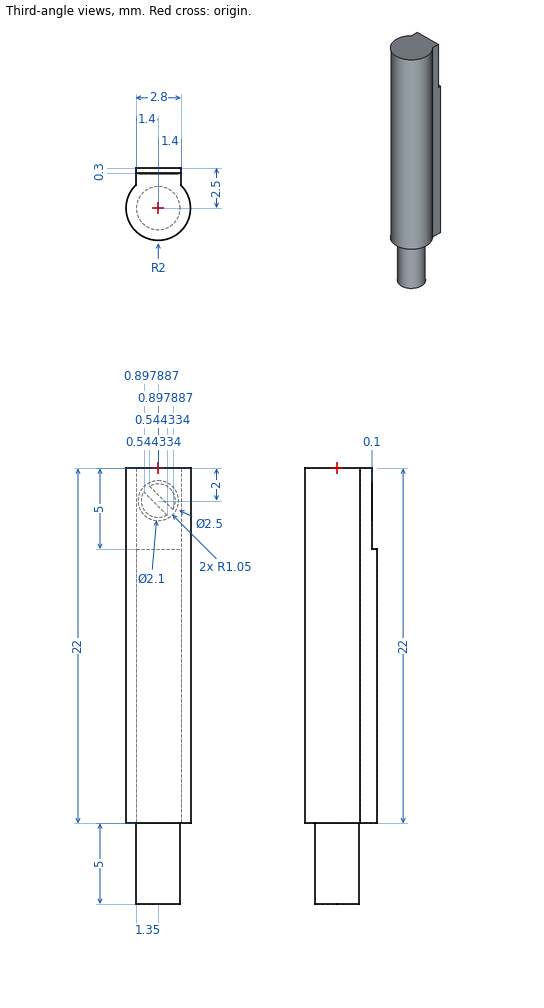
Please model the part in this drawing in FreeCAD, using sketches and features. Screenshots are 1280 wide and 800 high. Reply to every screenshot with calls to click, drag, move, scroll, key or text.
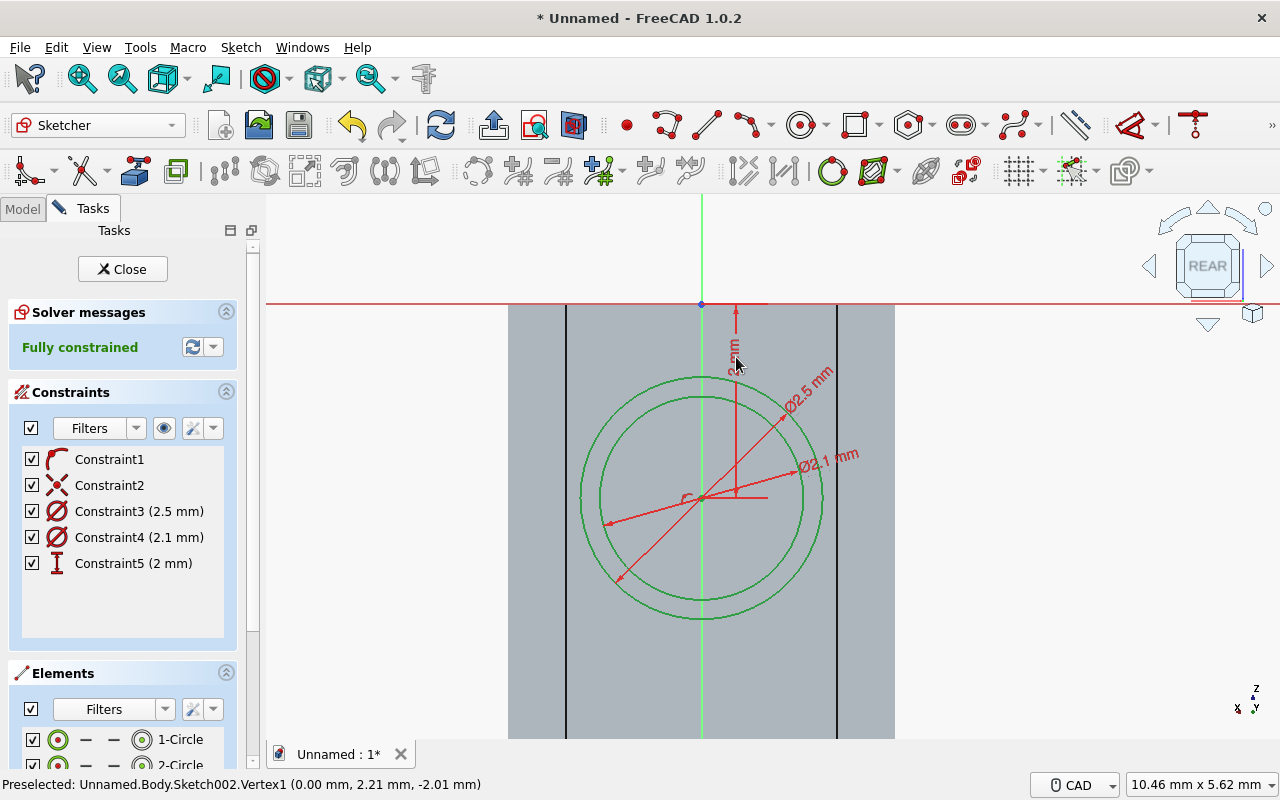
click(123, 269)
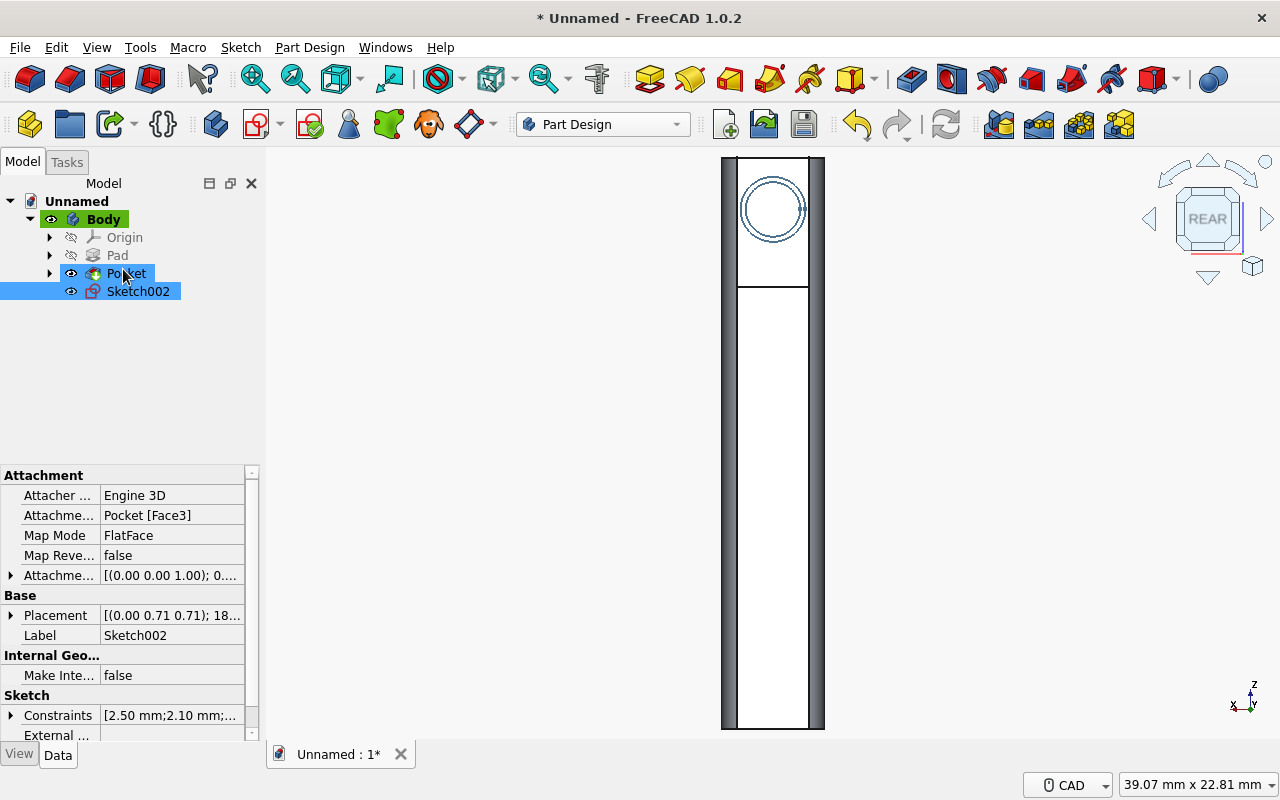
click(912, 80)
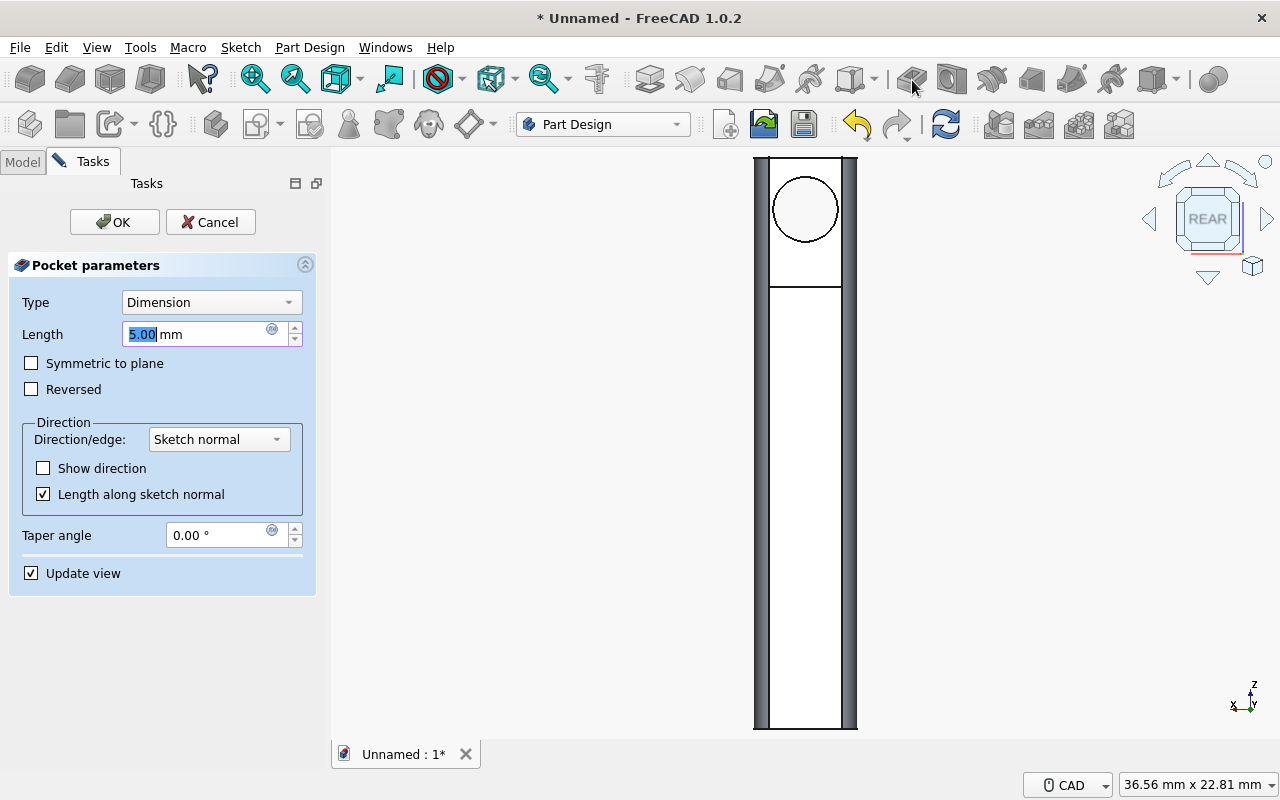
text(0.1)
key(Tab)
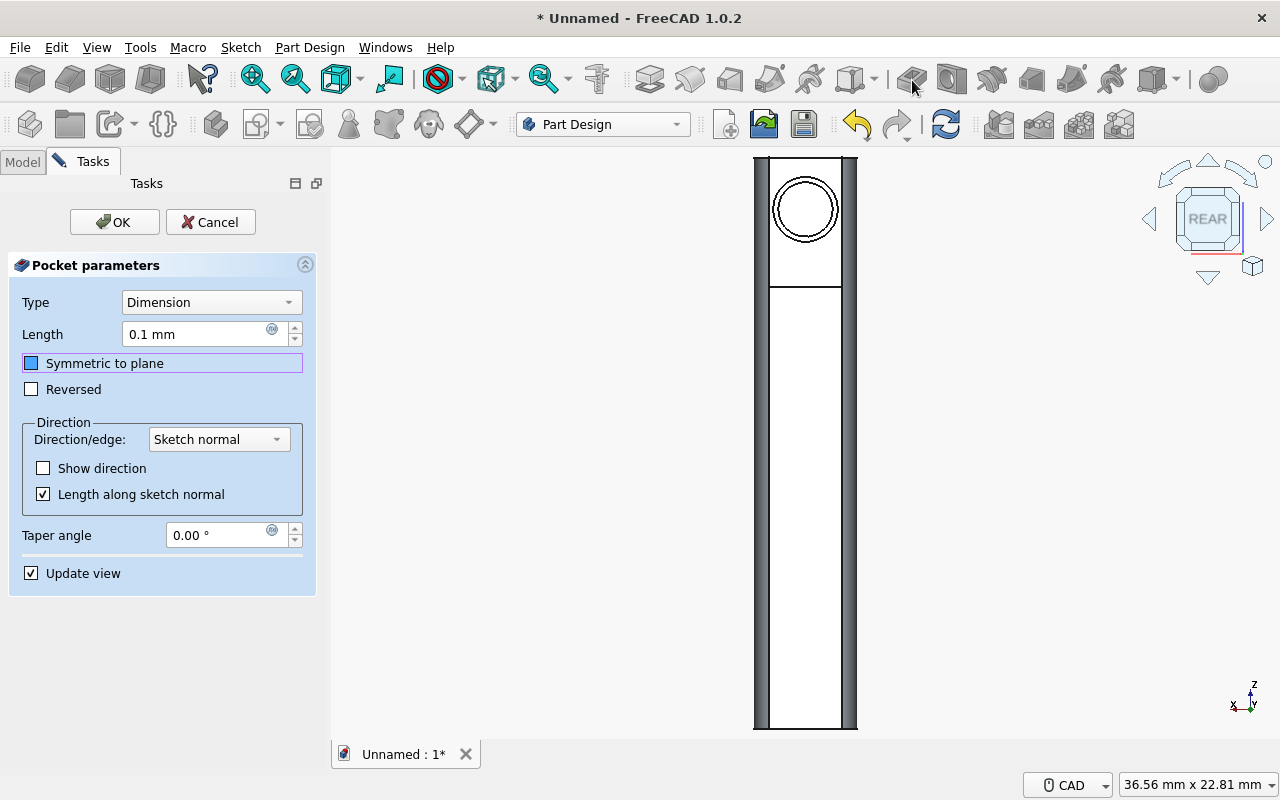
click(115, 222)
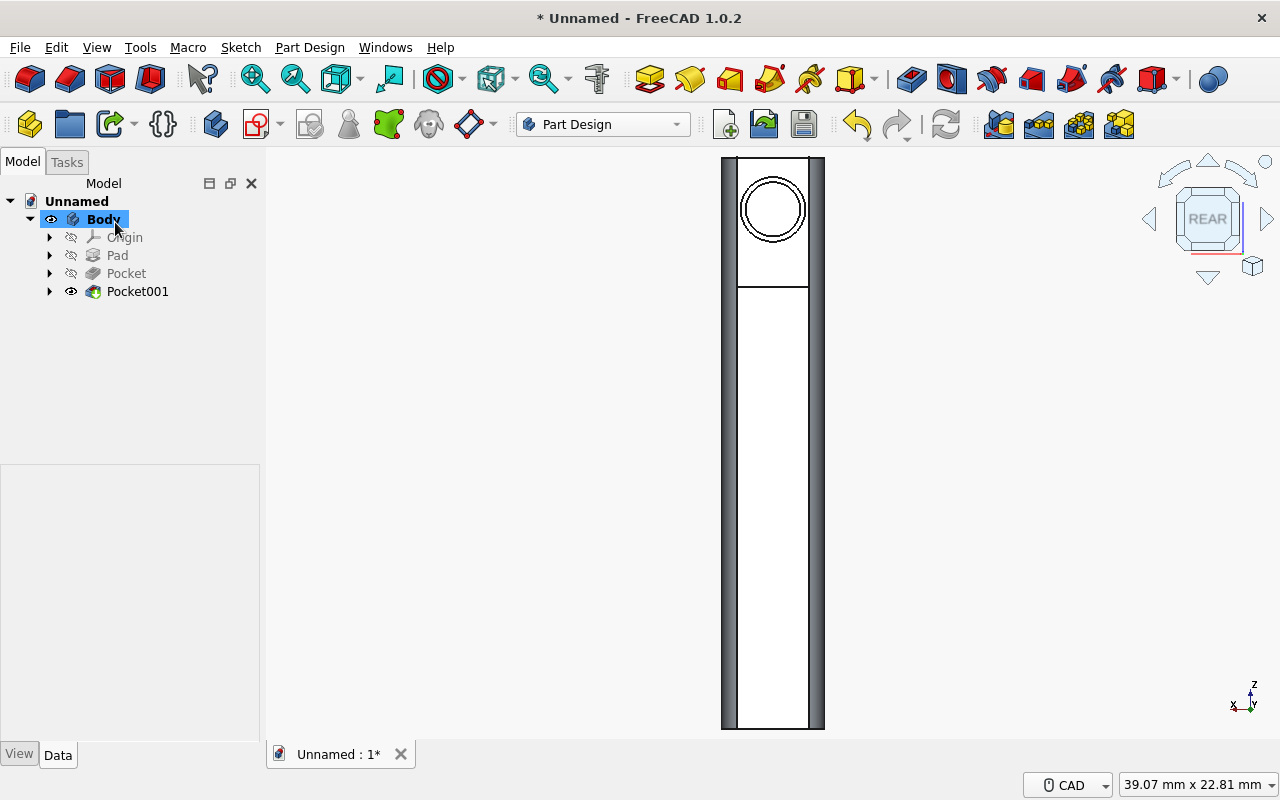
click(783, 258)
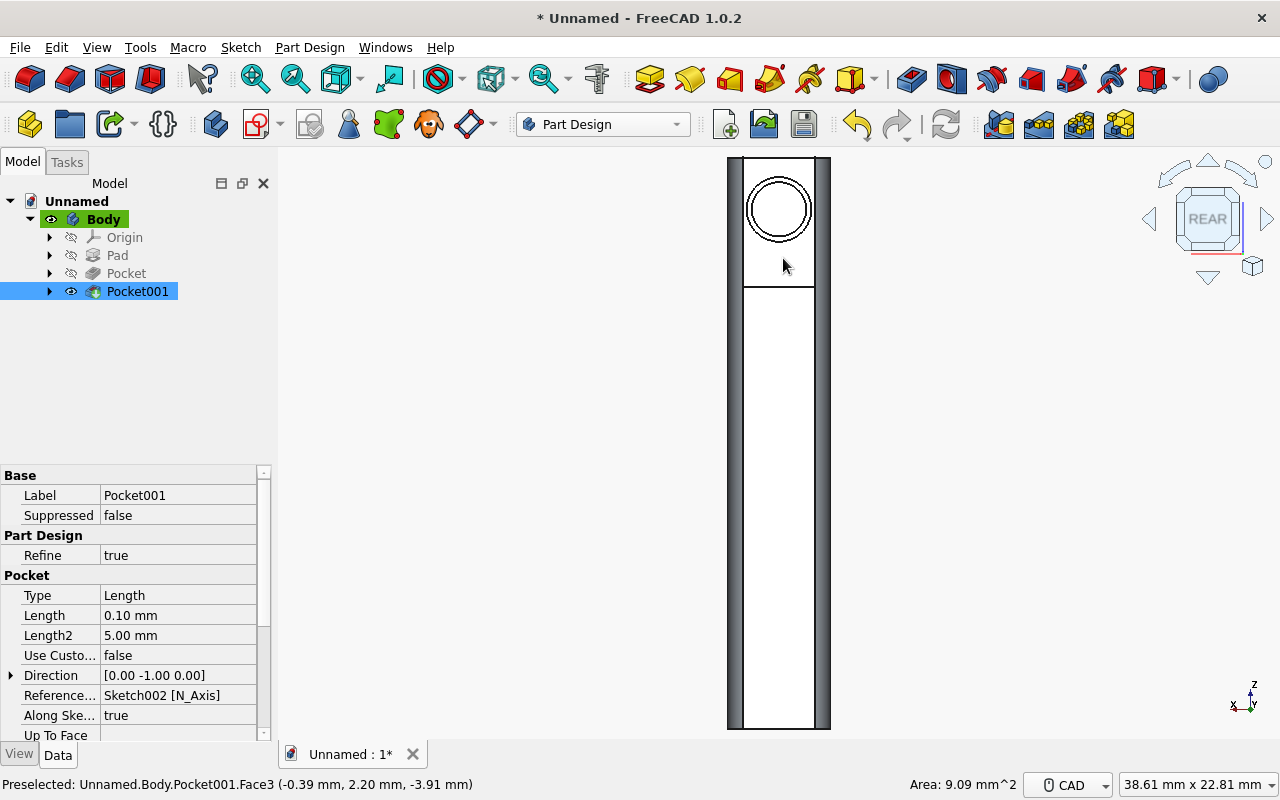
click(256, 124)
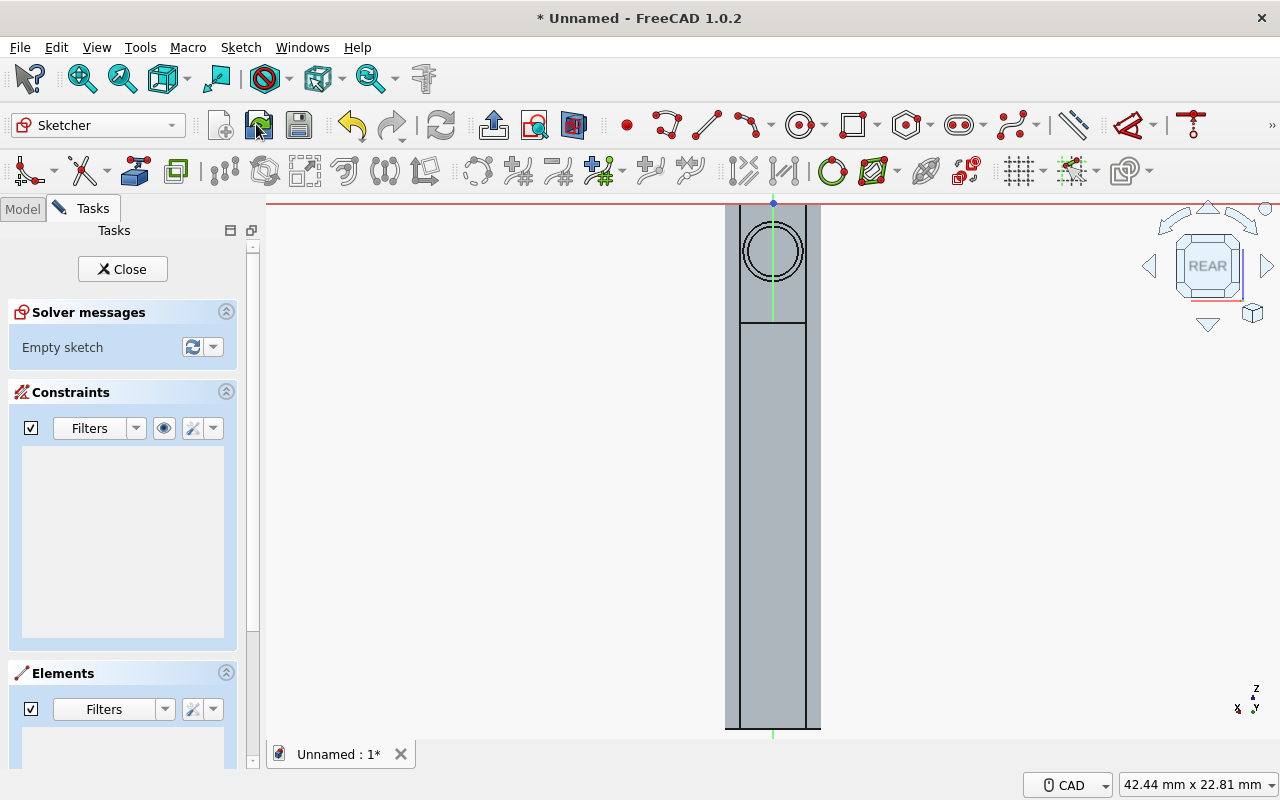
click(574, 126)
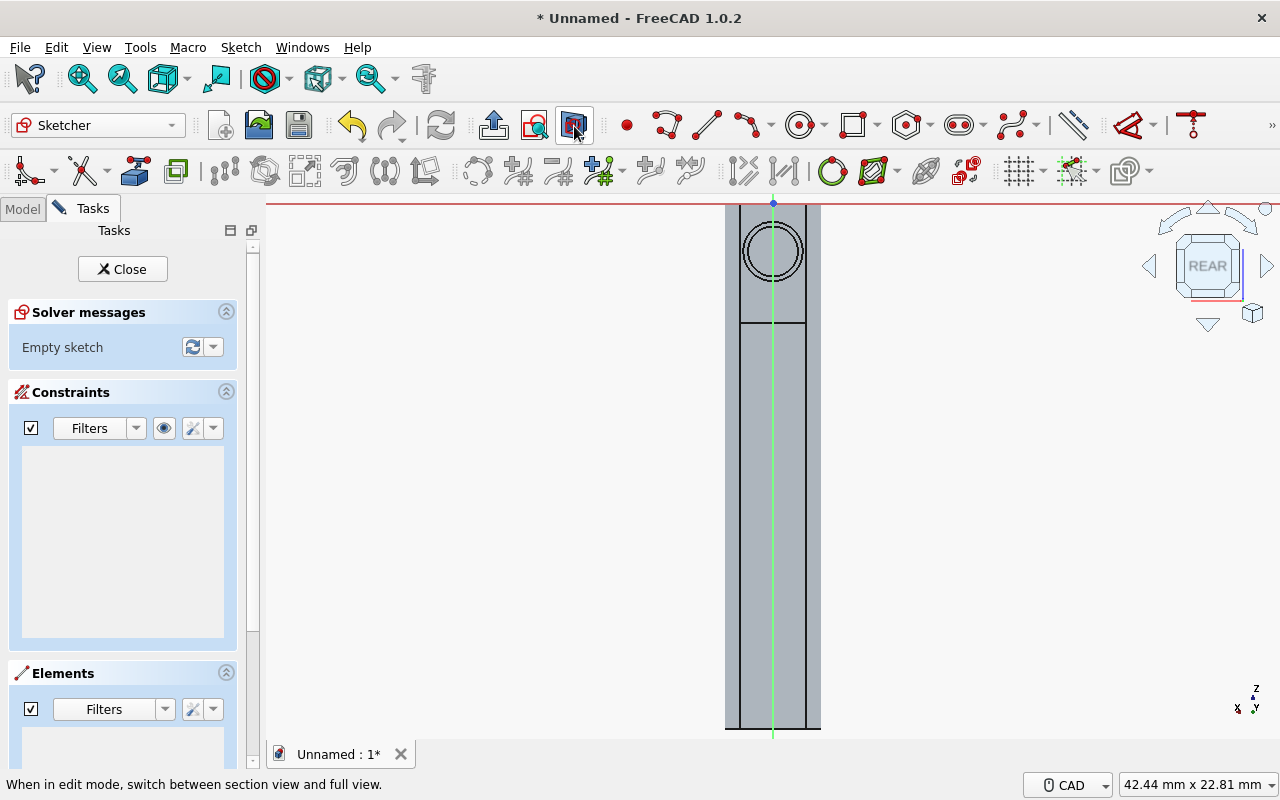
scroll(704, 466, down, 5)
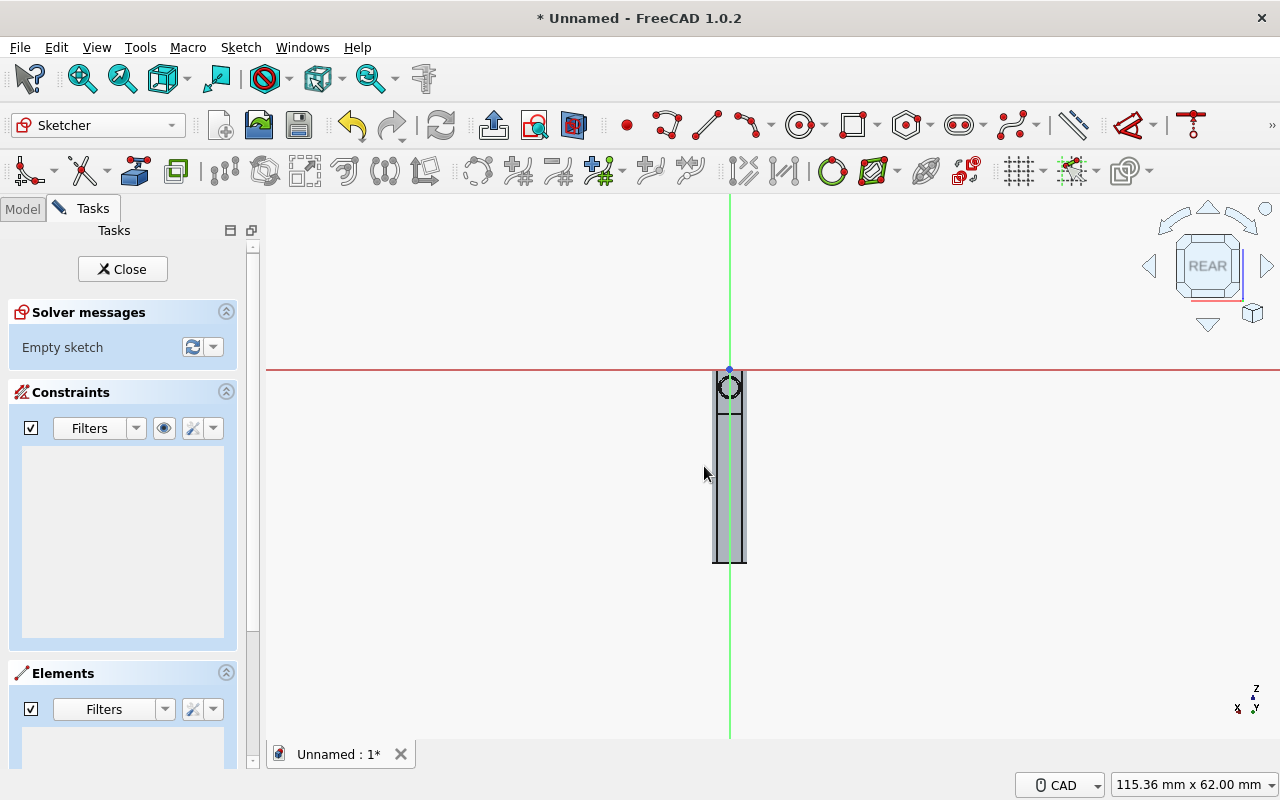
scroll(732, 376, up, 13)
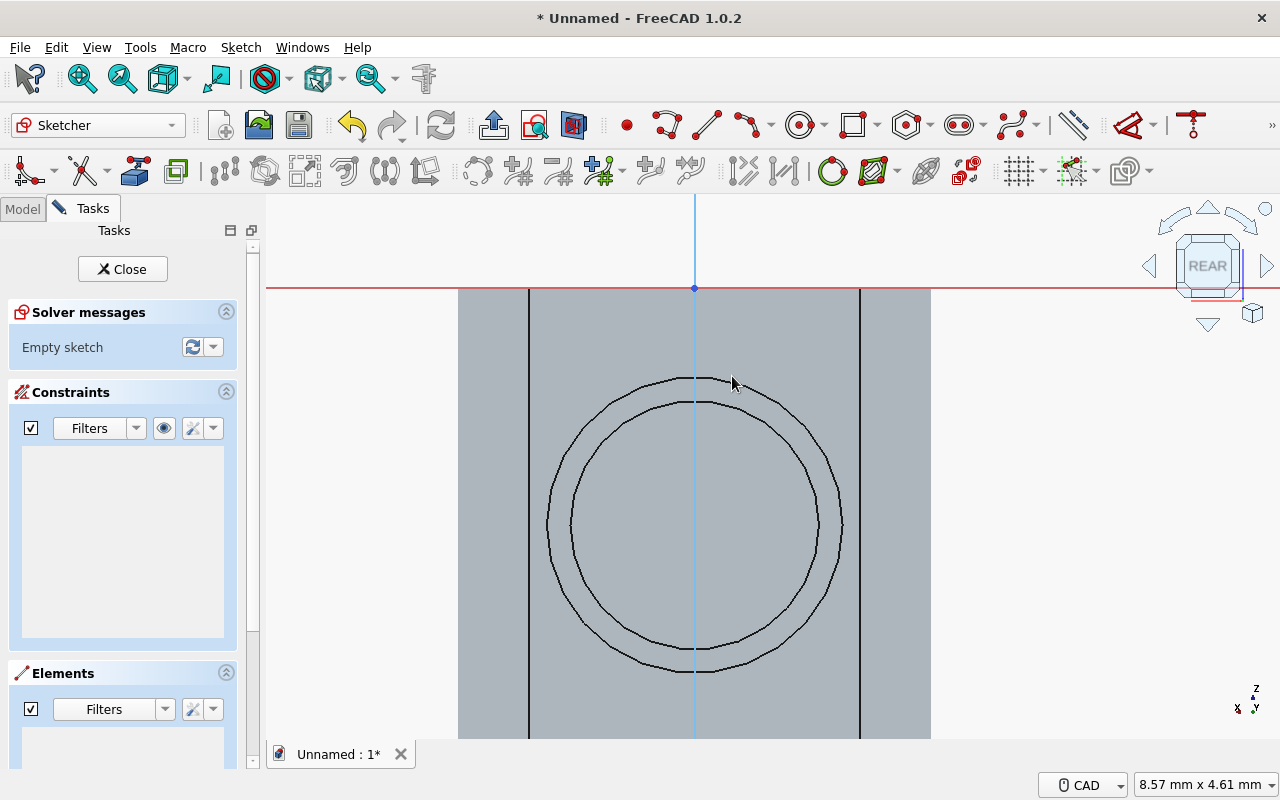
click(708, 126)